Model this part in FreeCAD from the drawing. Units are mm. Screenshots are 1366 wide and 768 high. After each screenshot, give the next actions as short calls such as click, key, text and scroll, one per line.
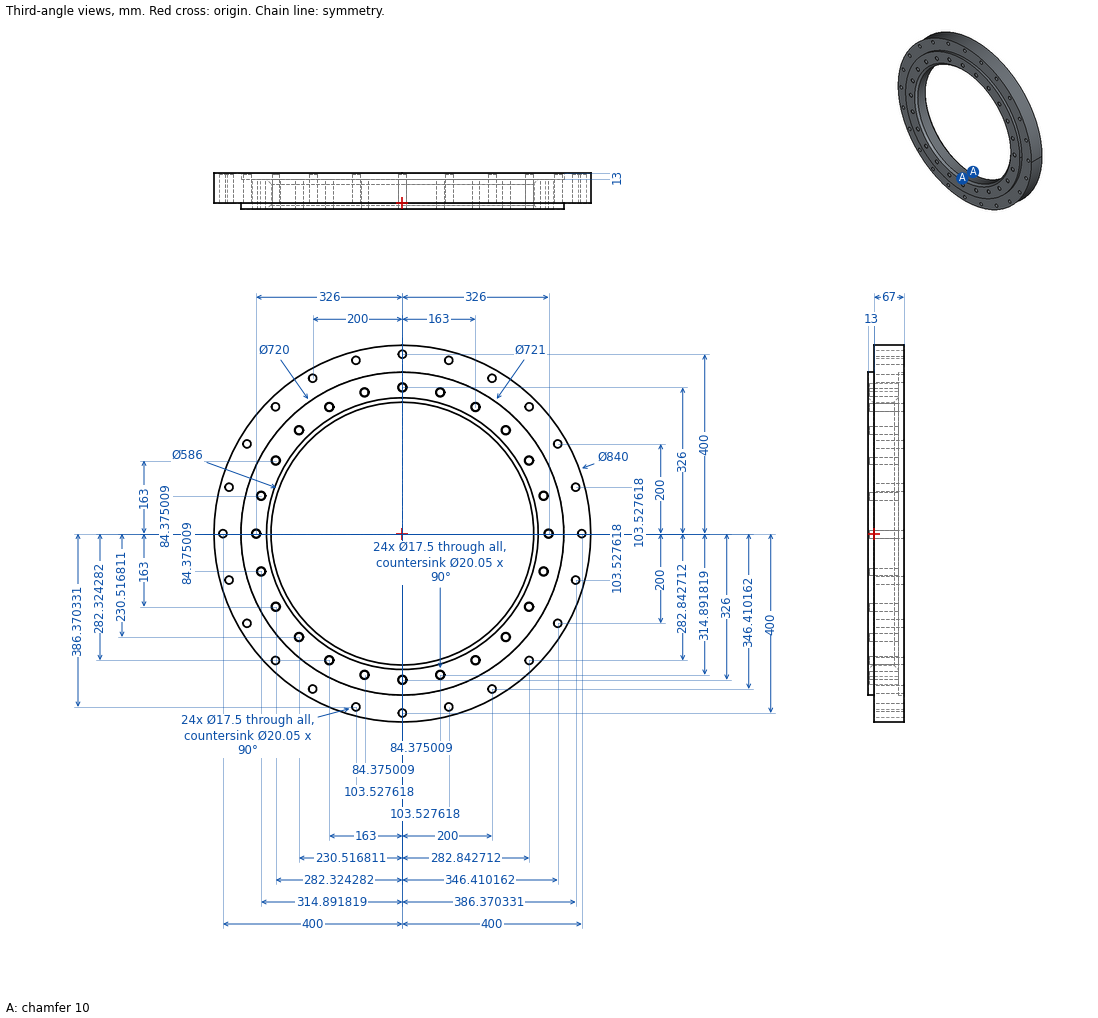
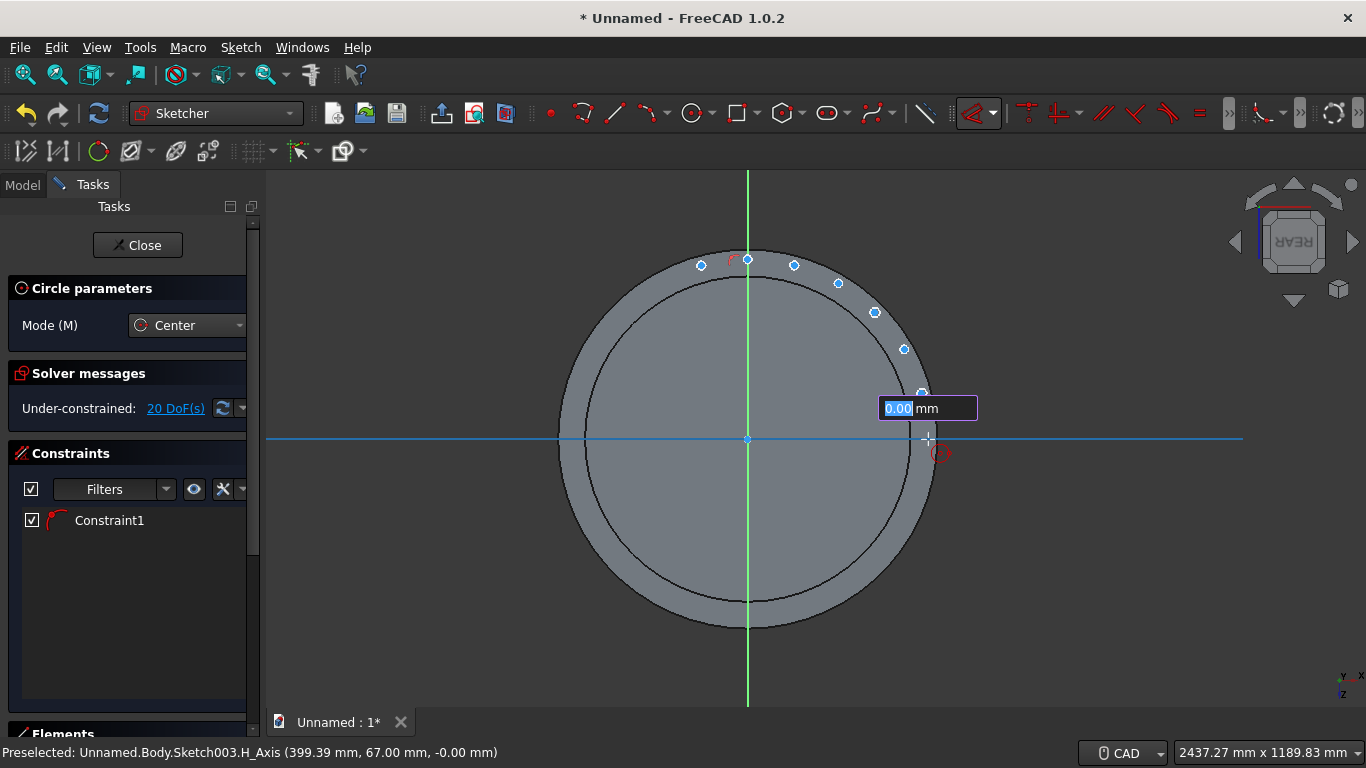
scroll(930, 435, up, 8)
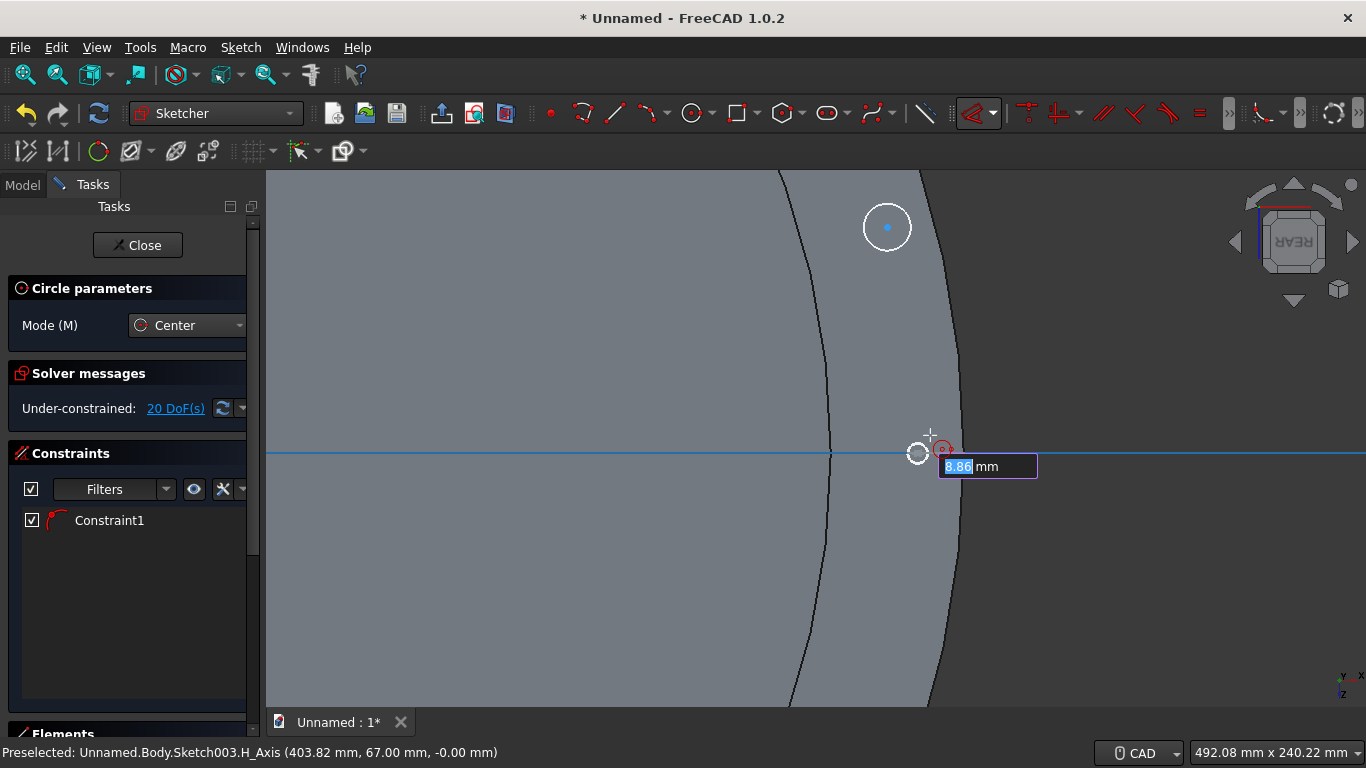
click(926, 435)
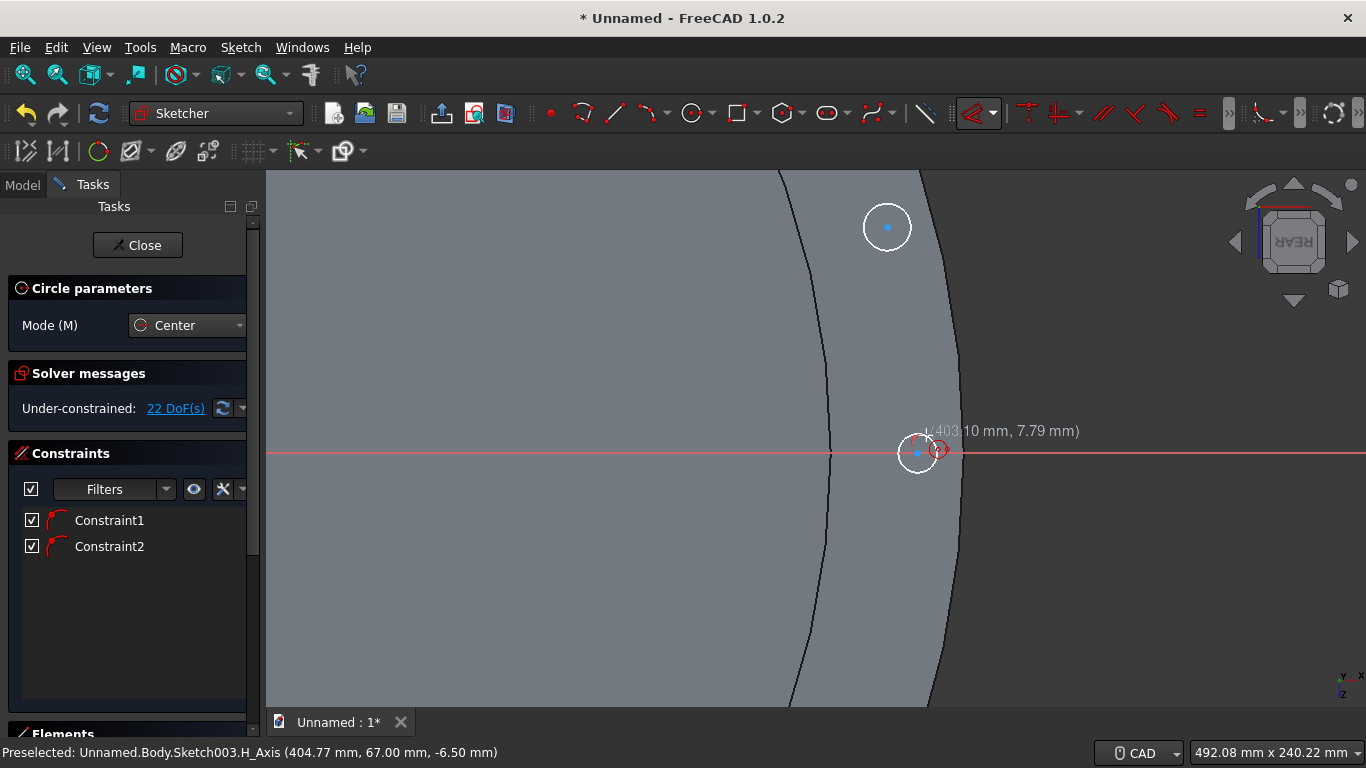
scroll(930, 435, down, 8)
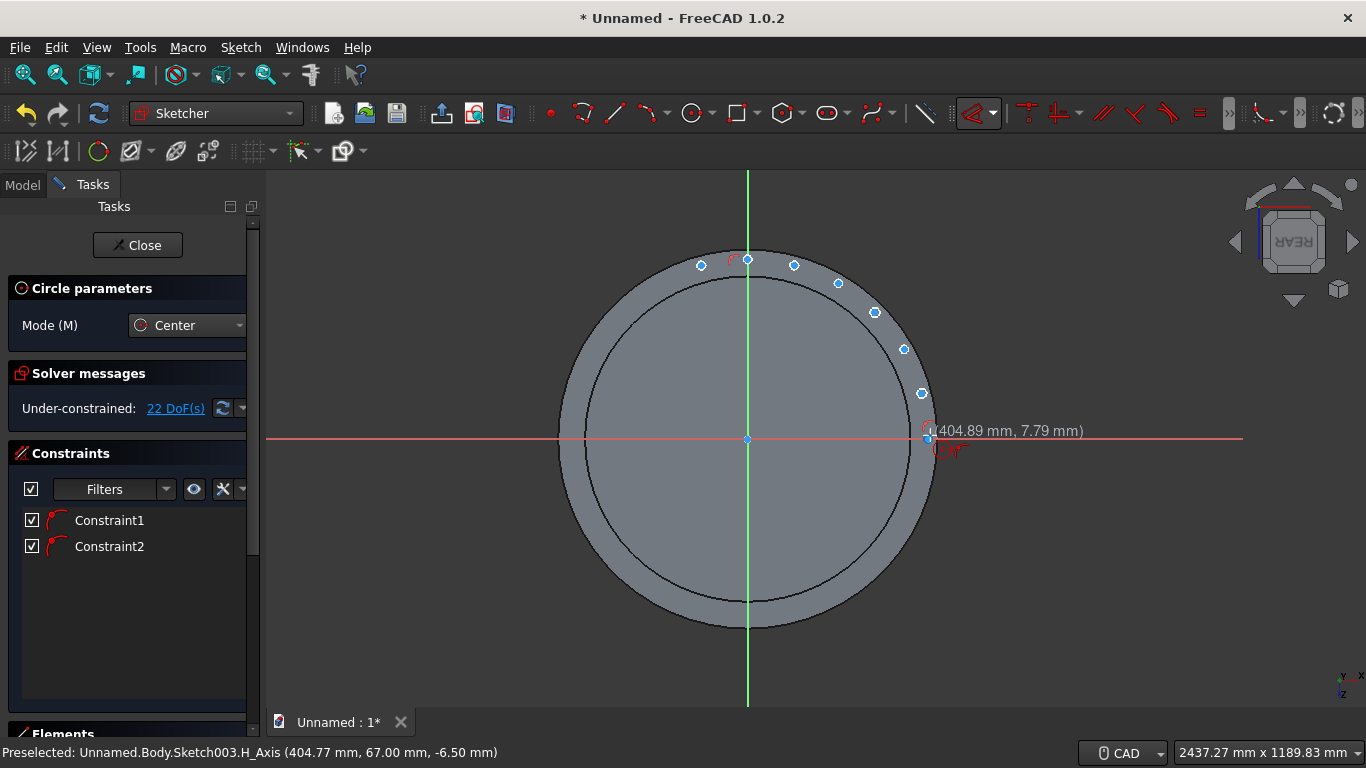
scroll(922, 486, up, 9)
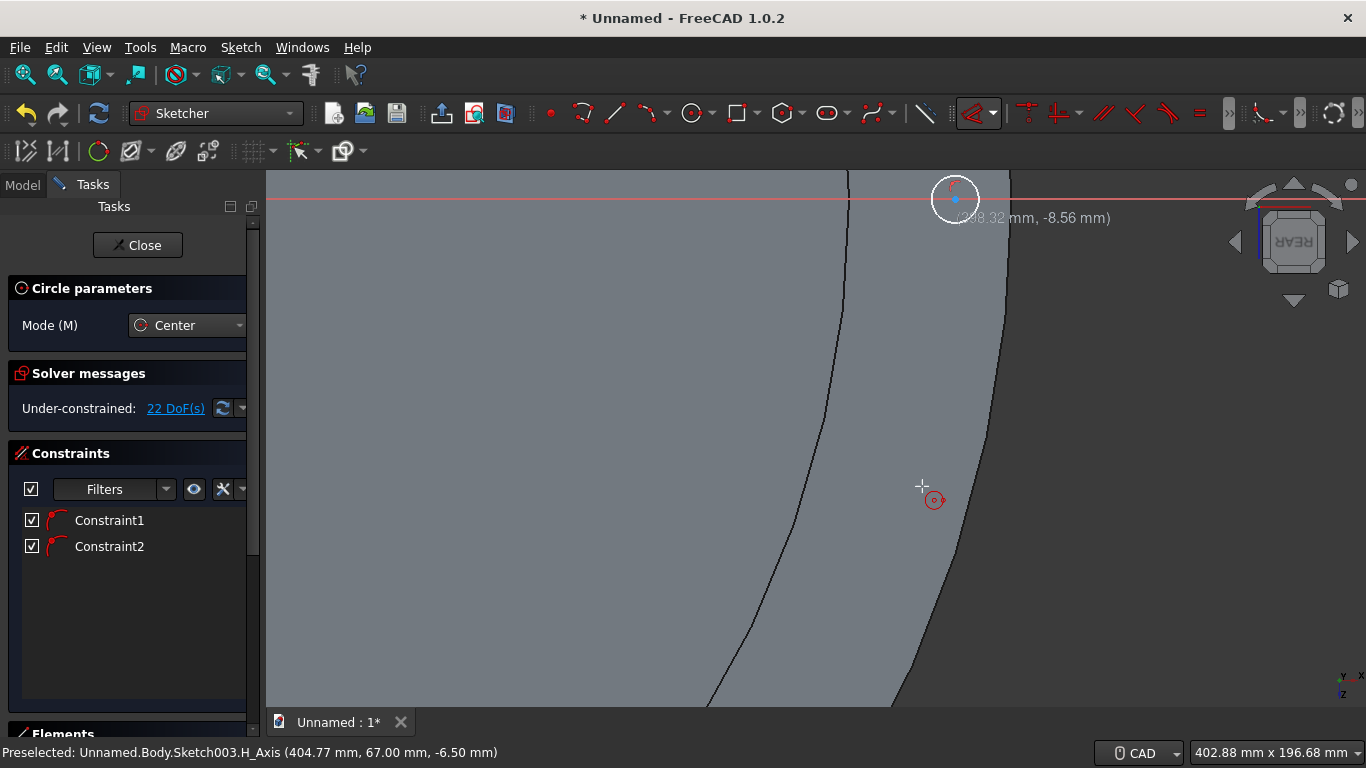
scroll(922, 486, down, 9)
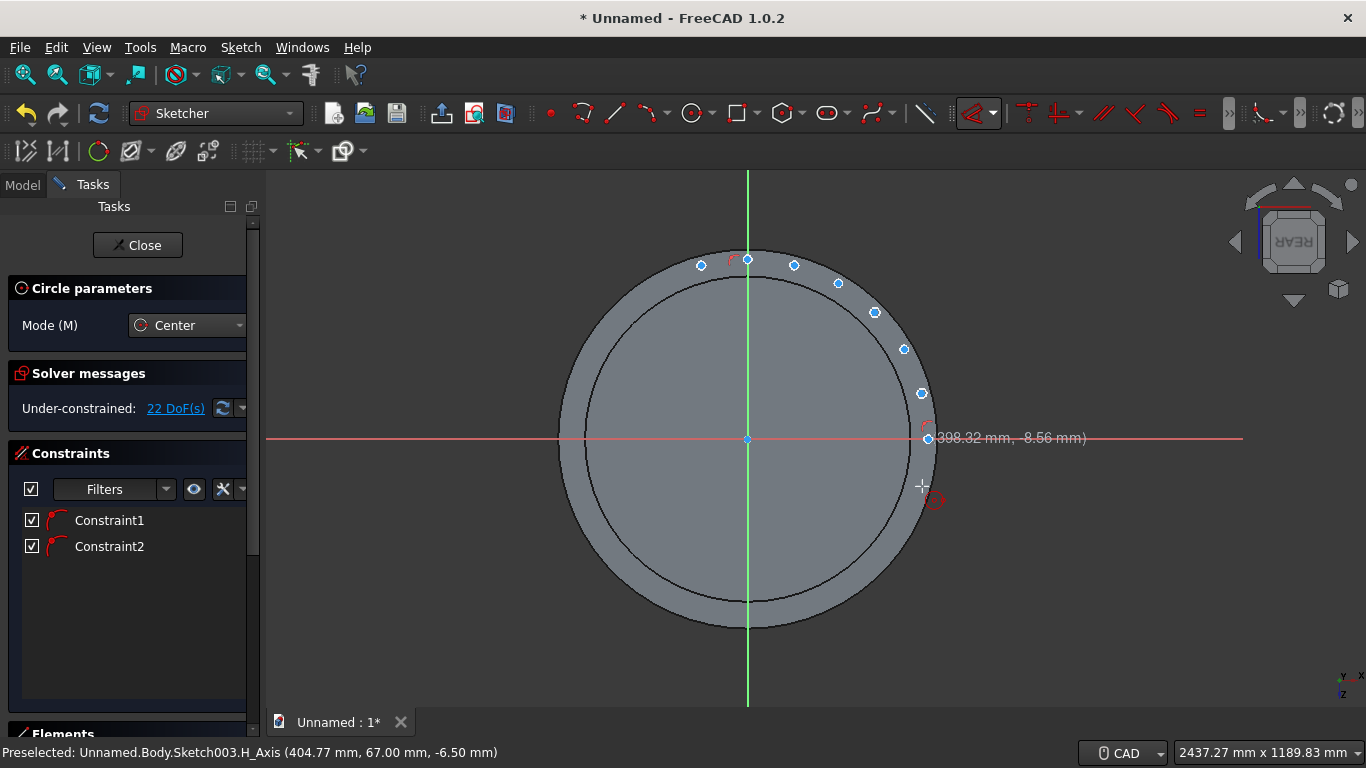
click(922, 486)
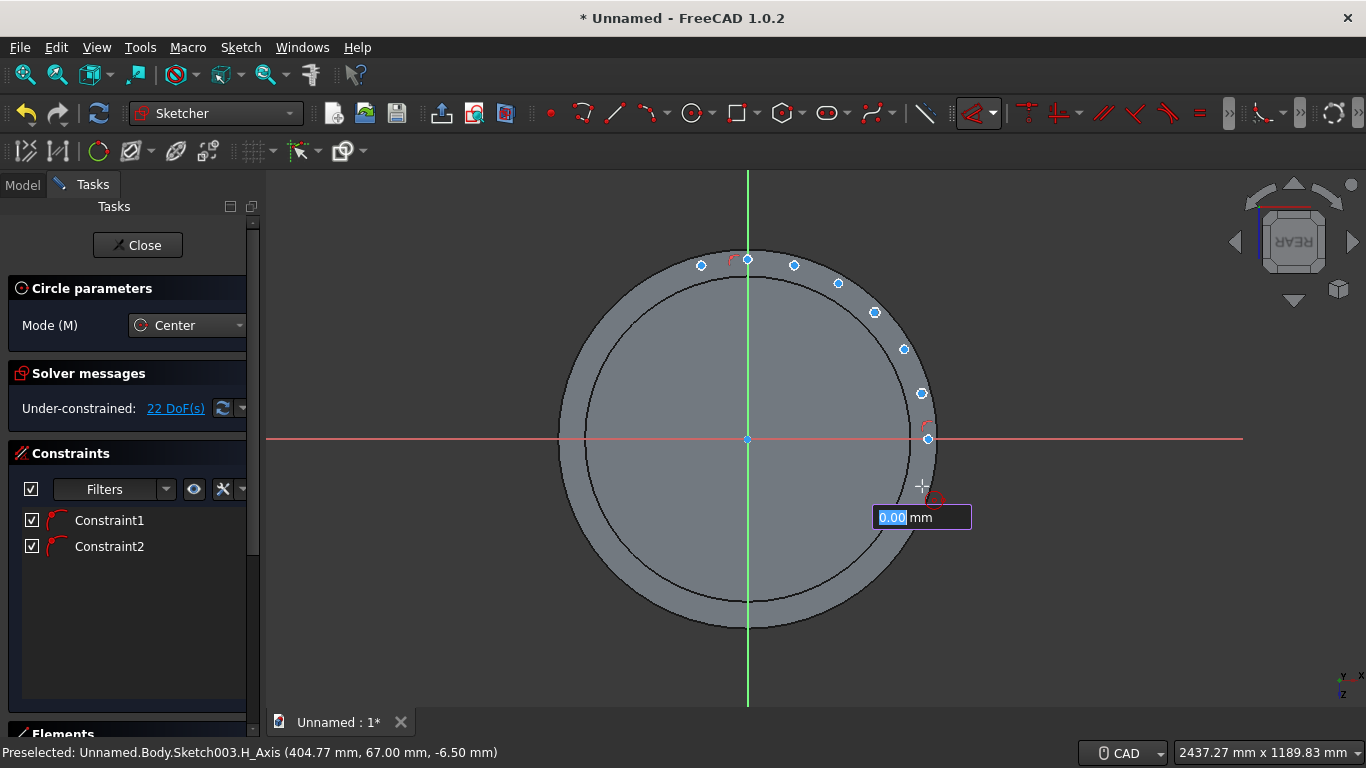
scroll(925, 483, up, 7)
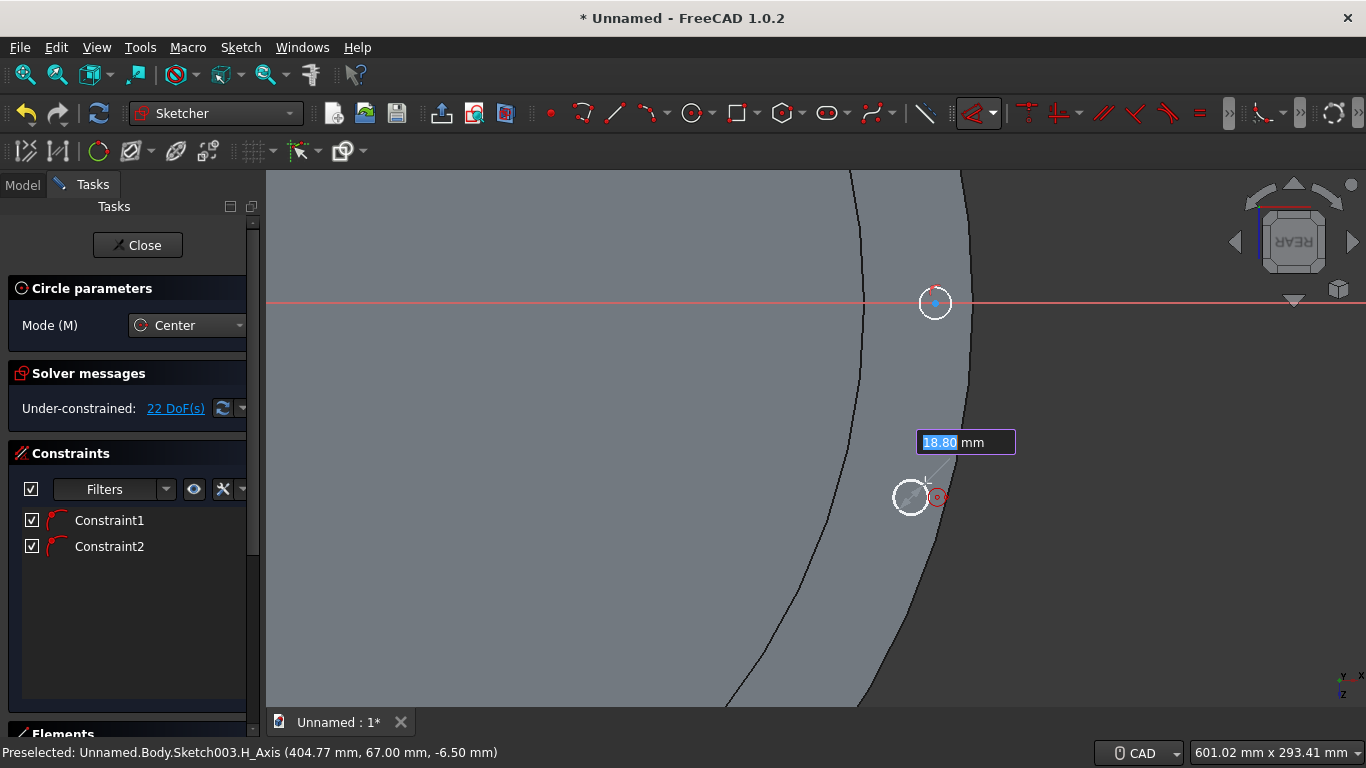
click(923, 481)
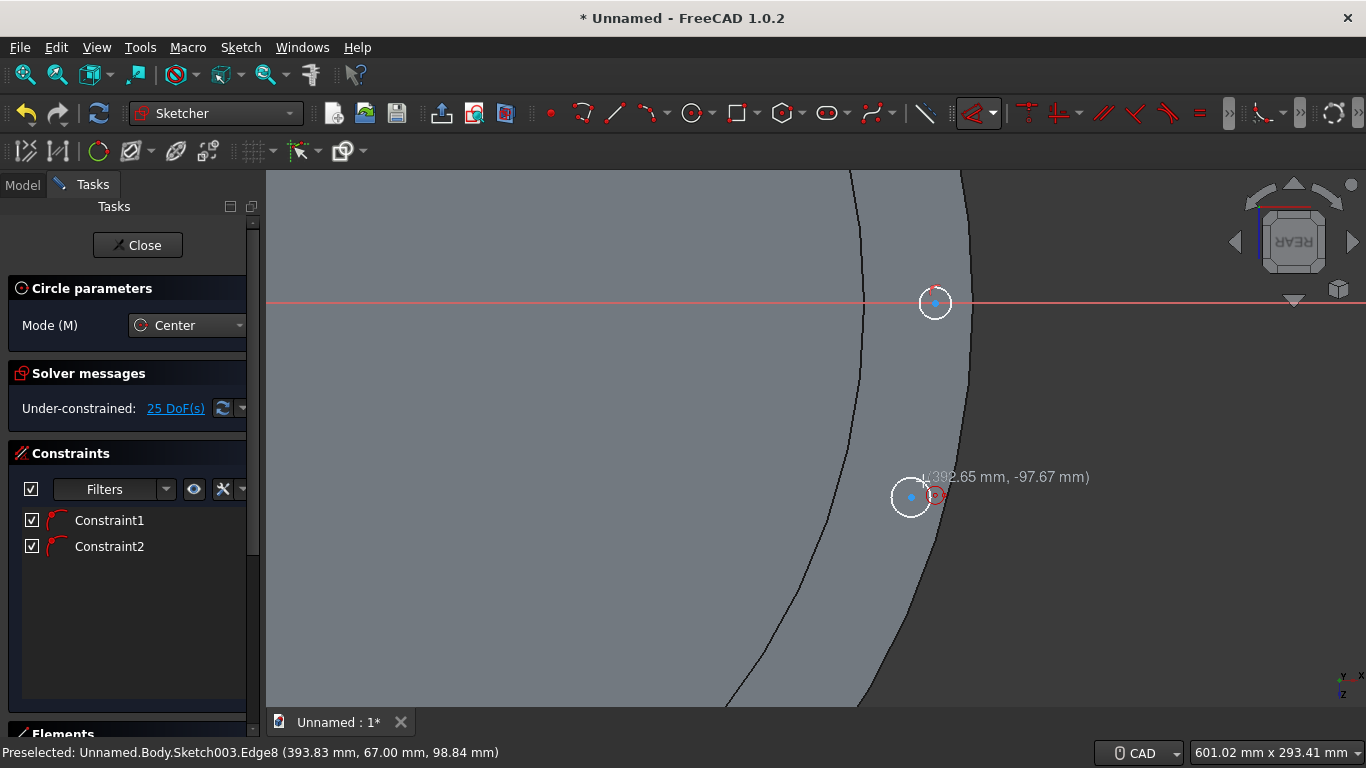
scroll(838, 669, up, 2)